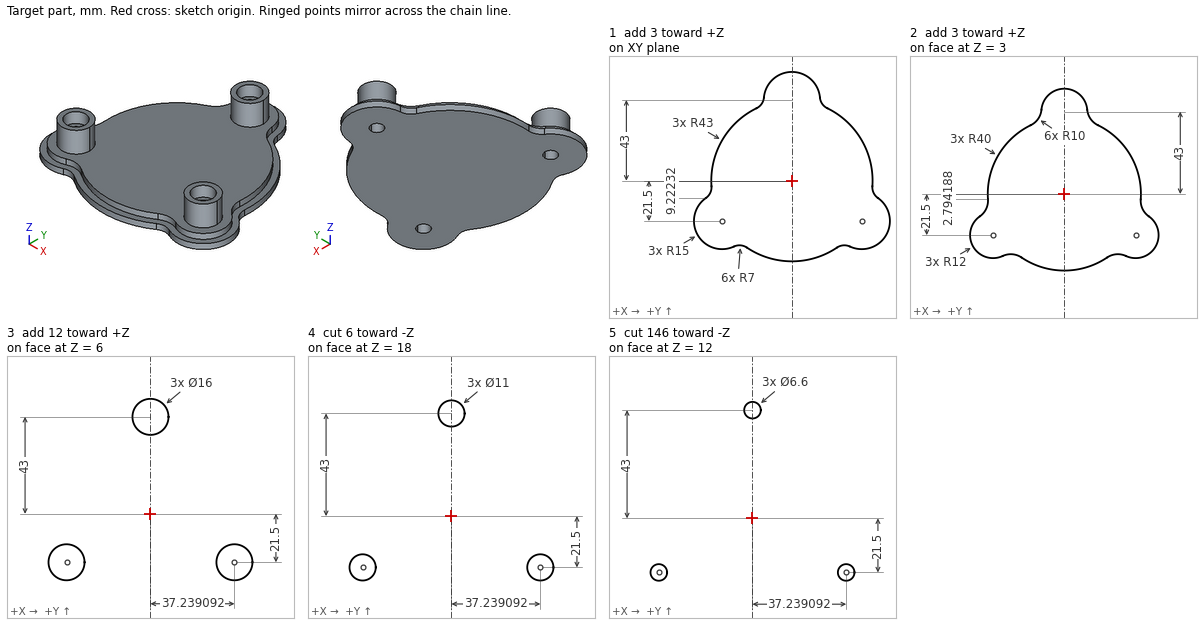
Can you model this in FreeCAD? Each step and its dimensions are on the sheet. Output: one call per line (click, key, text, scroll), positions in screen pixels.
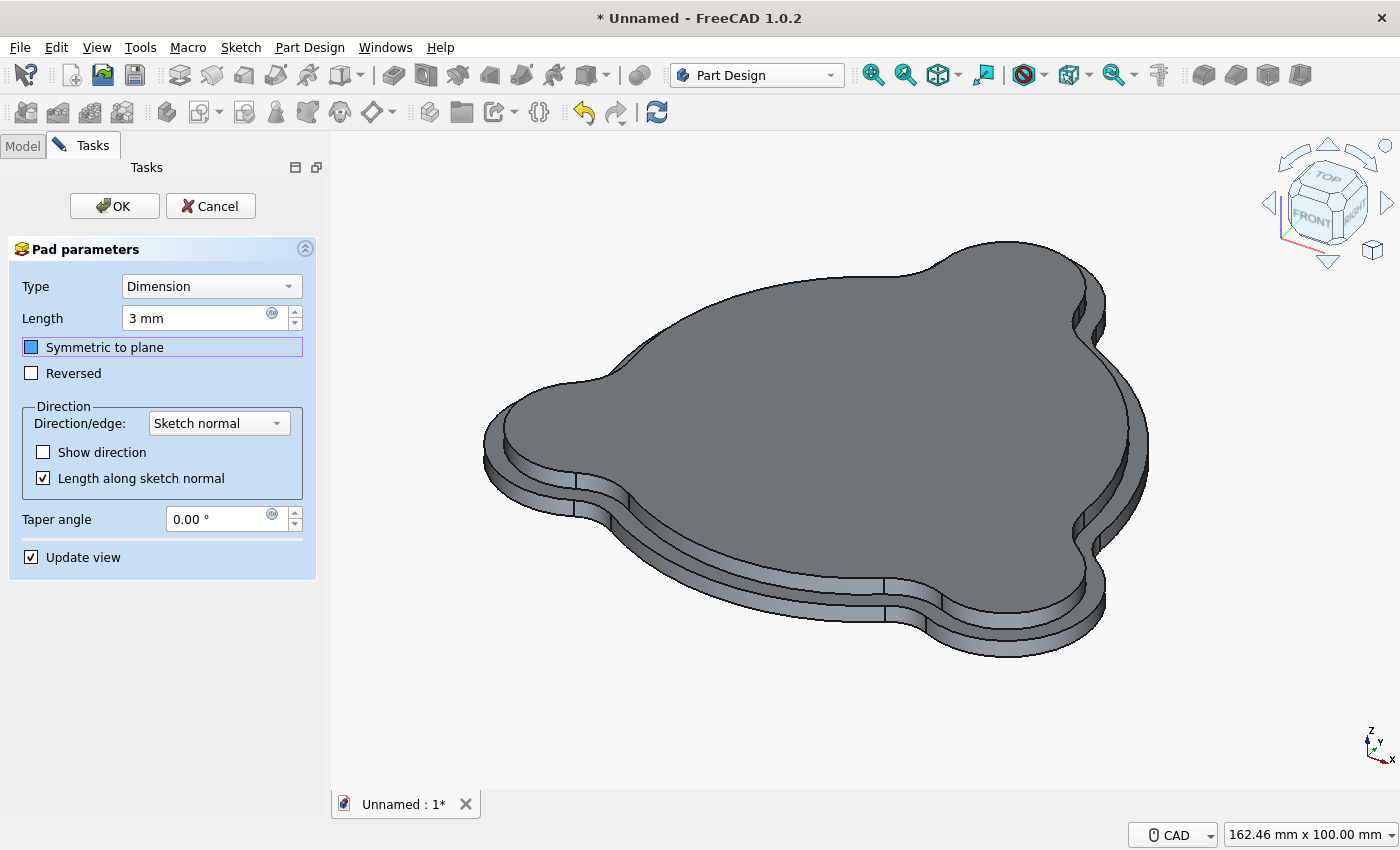
click(115, 206)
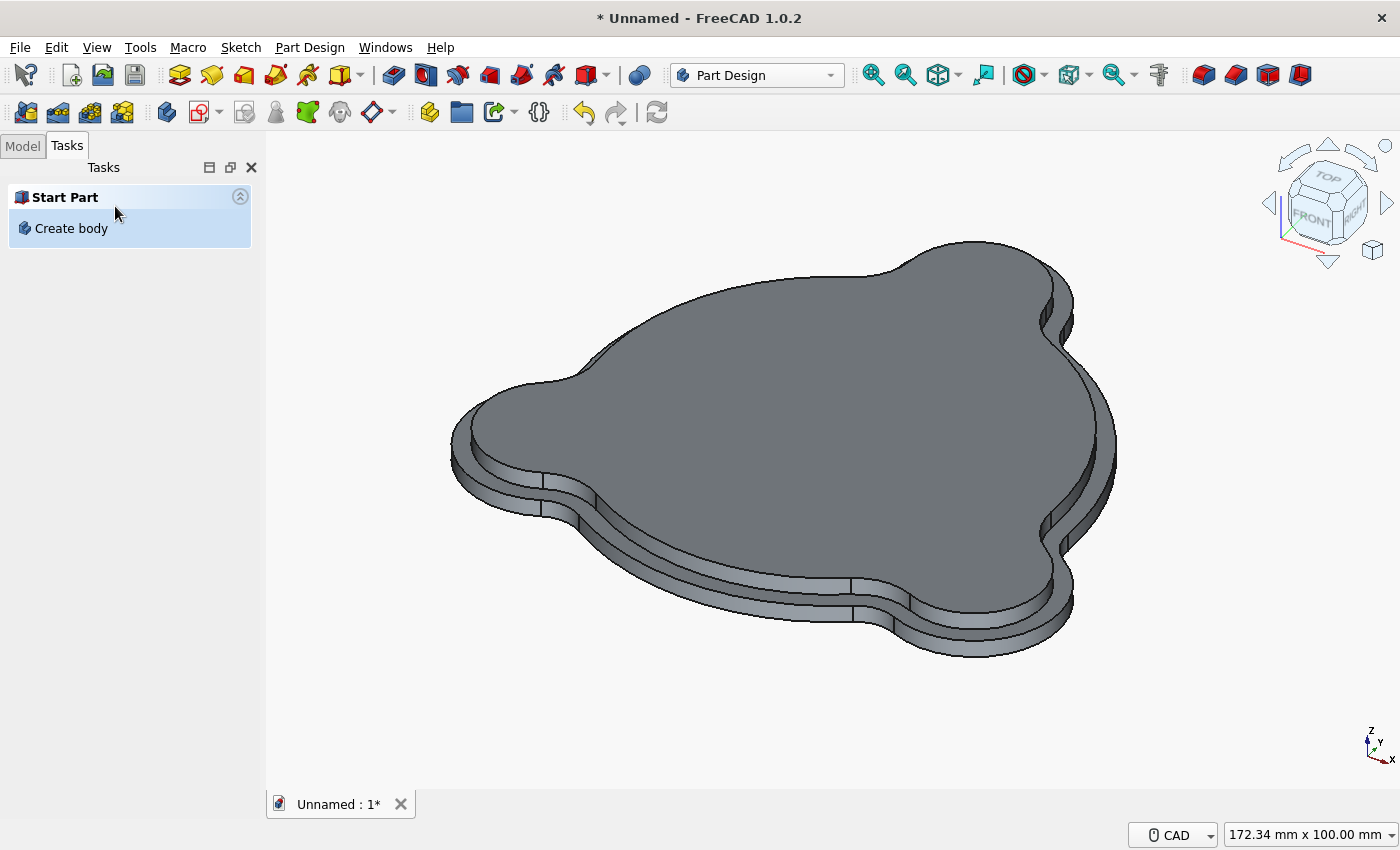
click(813, 447)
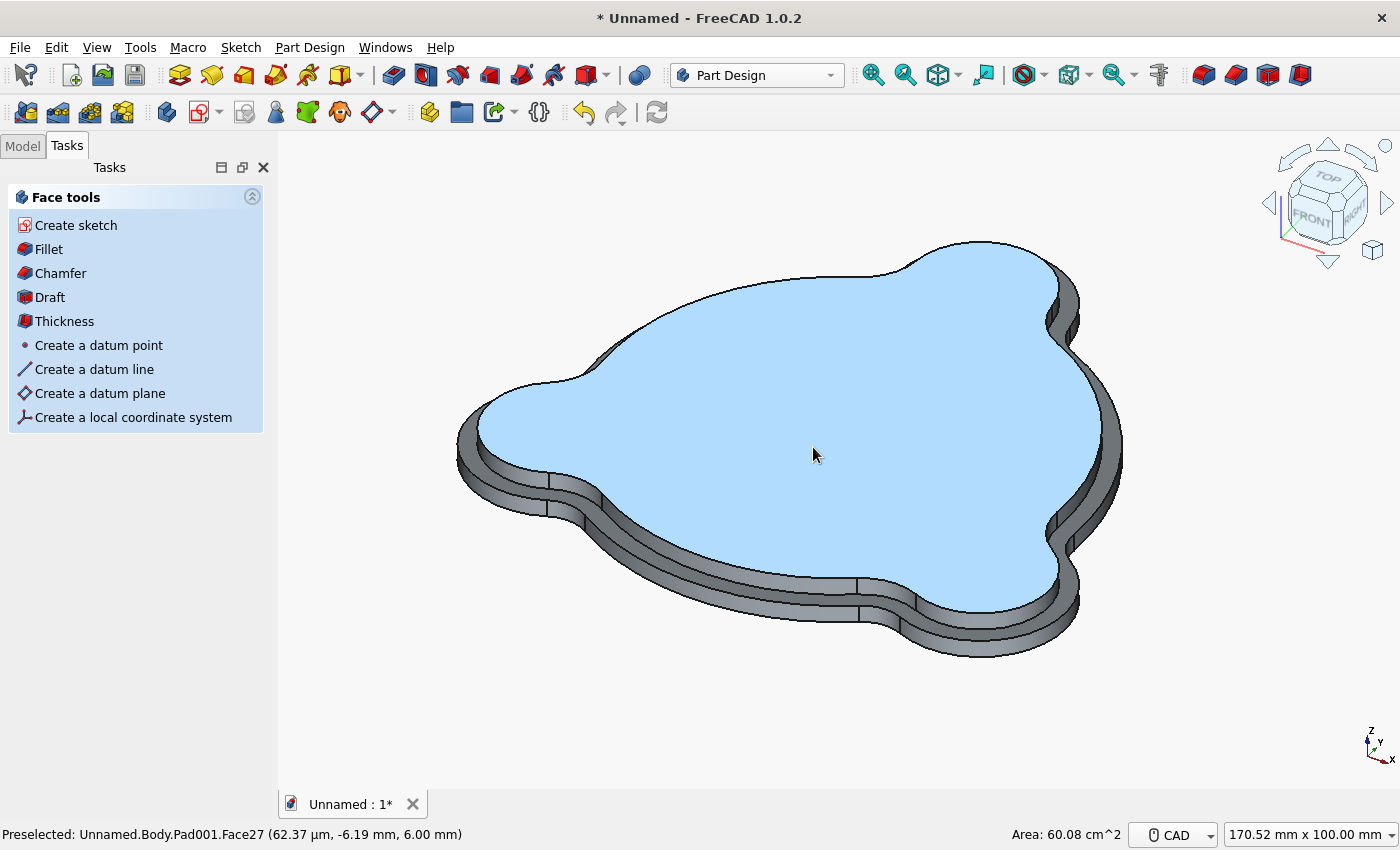
click(200, 112)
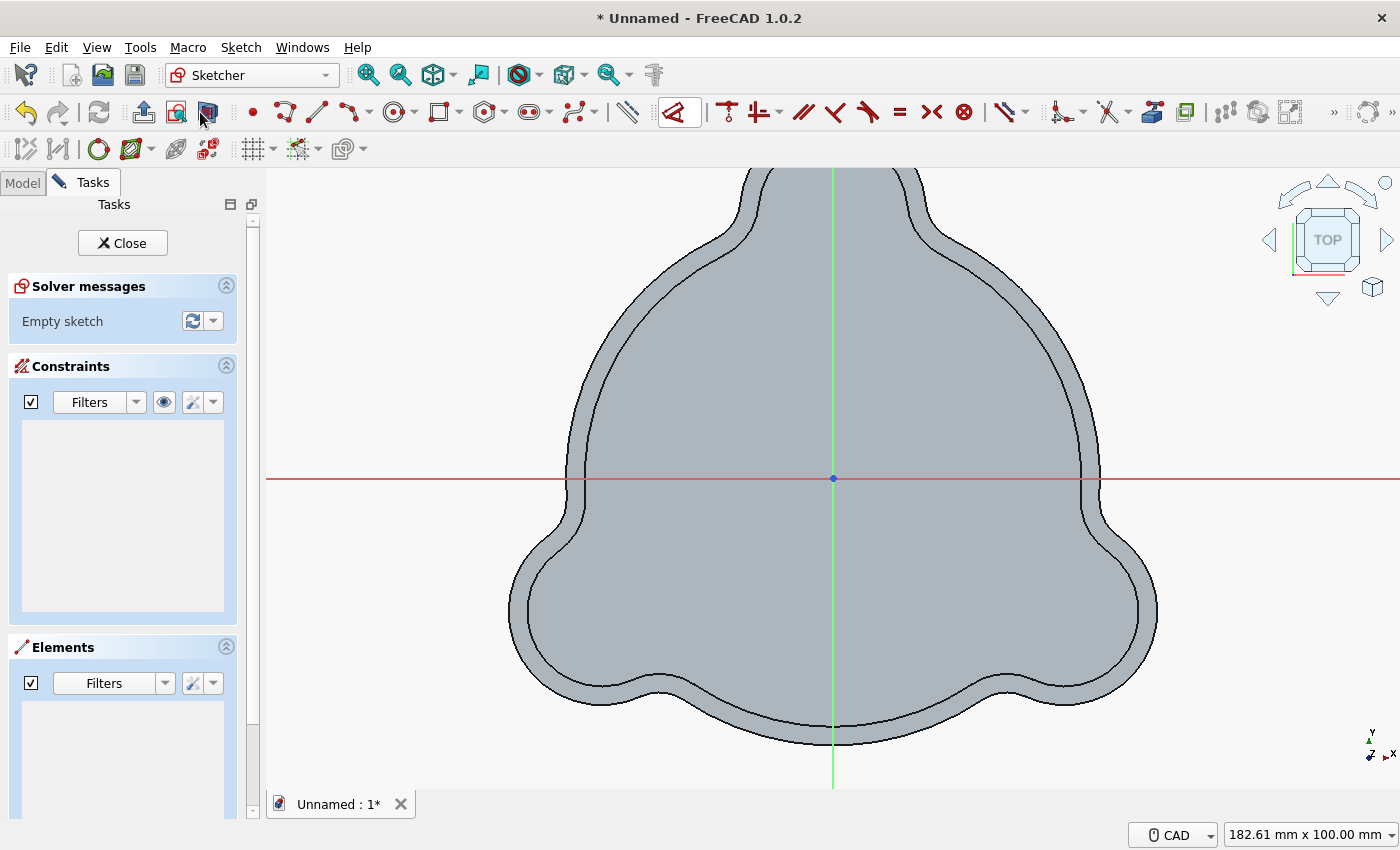
scroll(455, 761, down, 1)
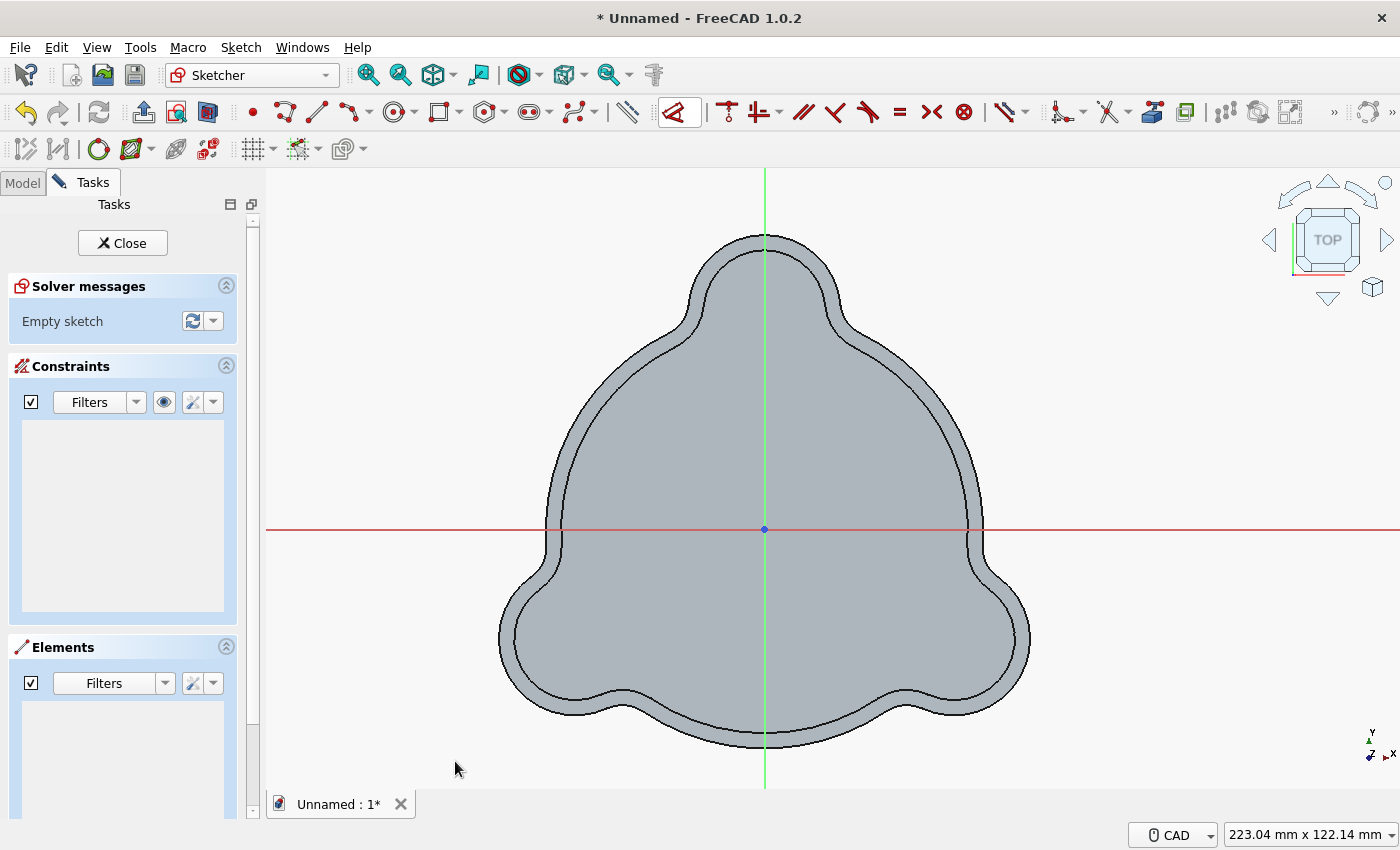
click(394, 112)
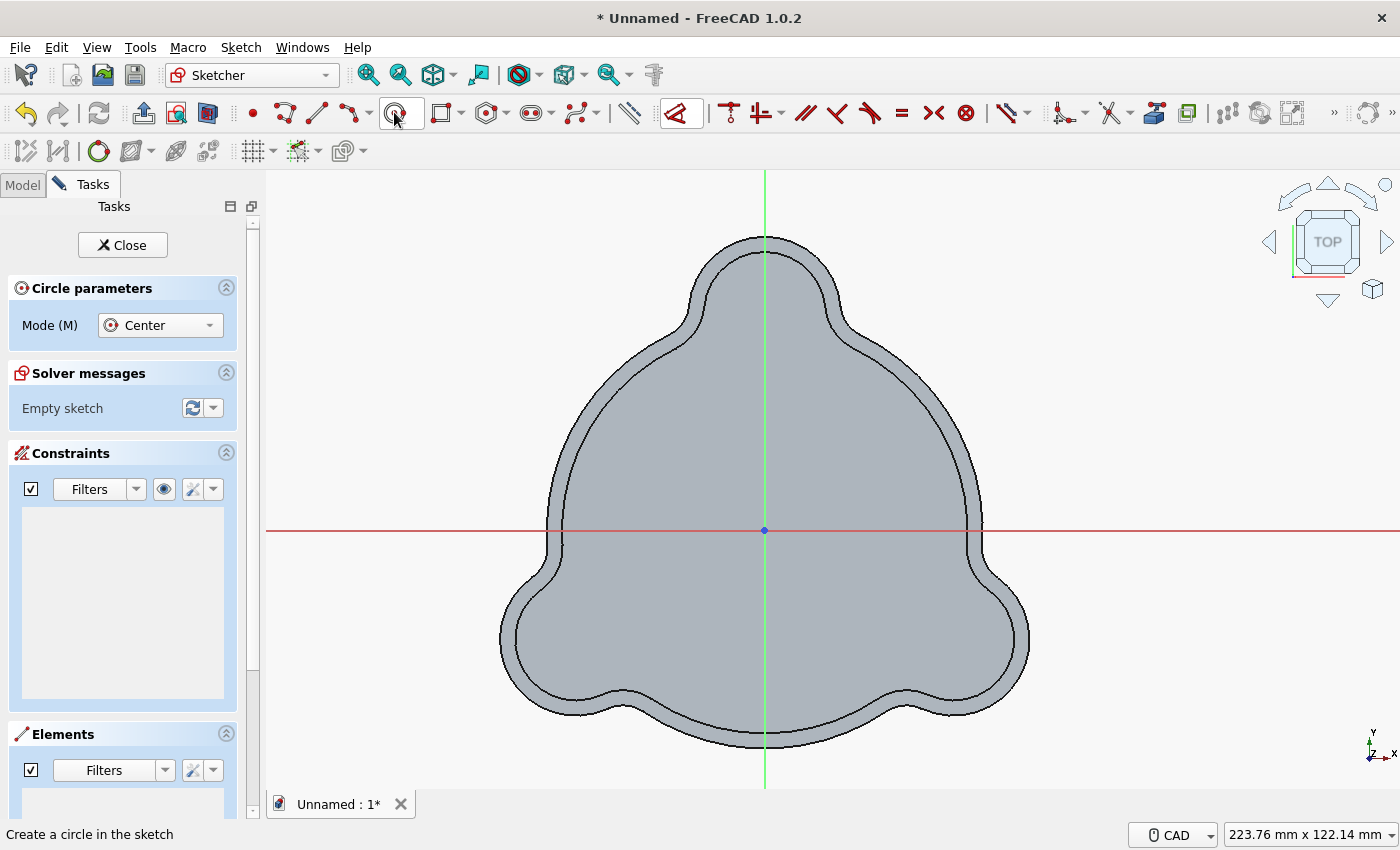
click(765, 313)
move(793, 284)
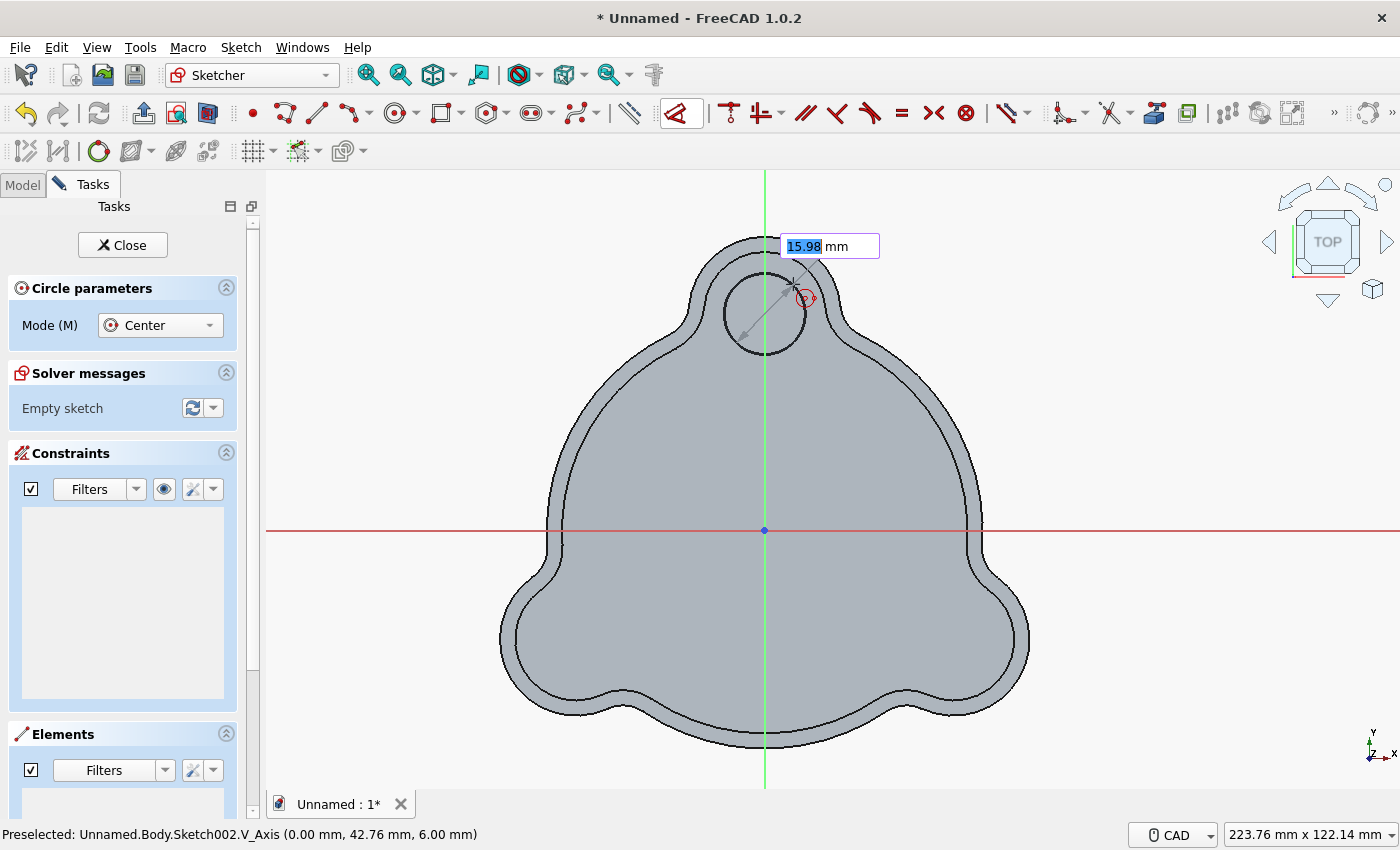
text(16)
key(Return)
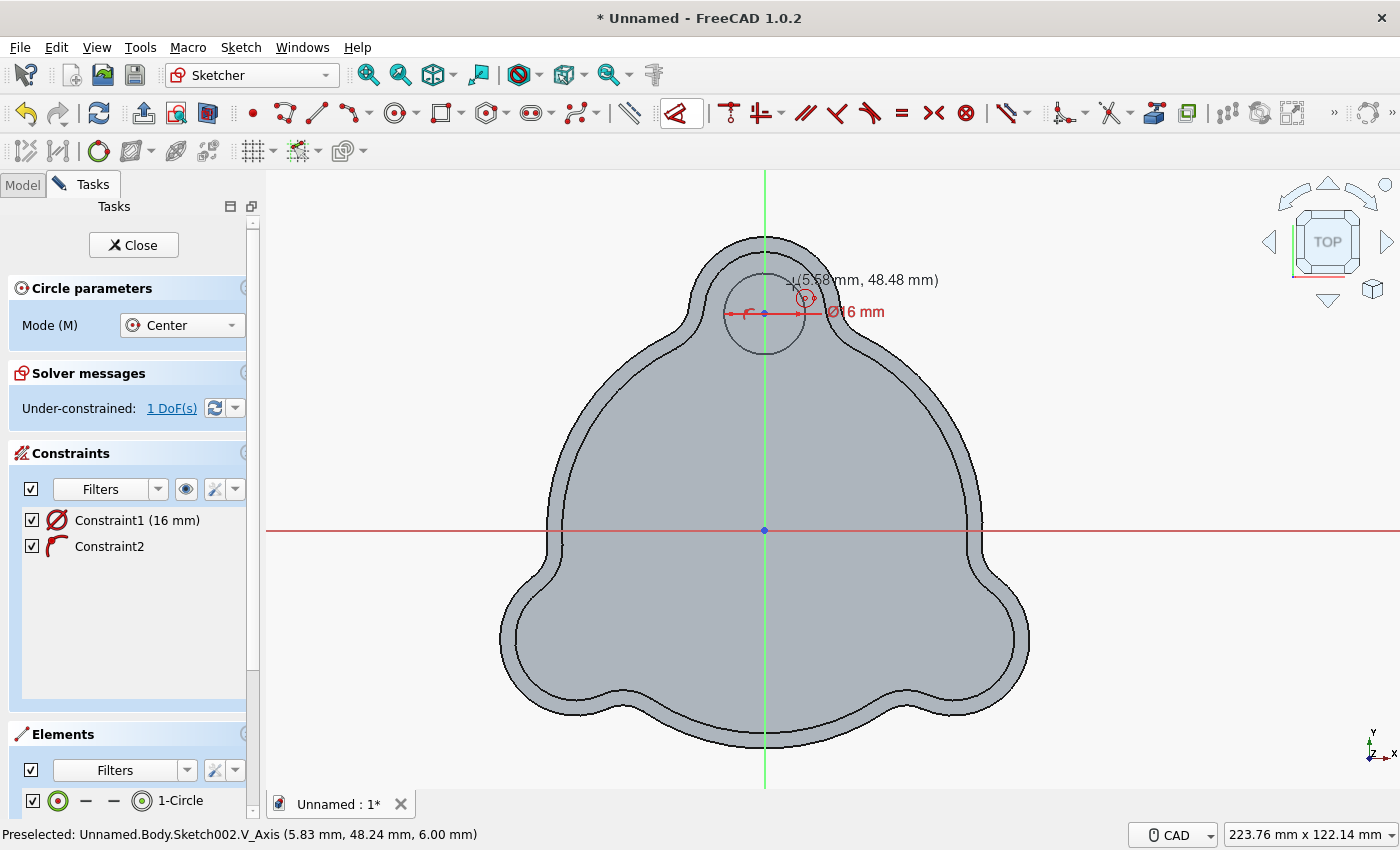
click(953, 640)
move(982, 611)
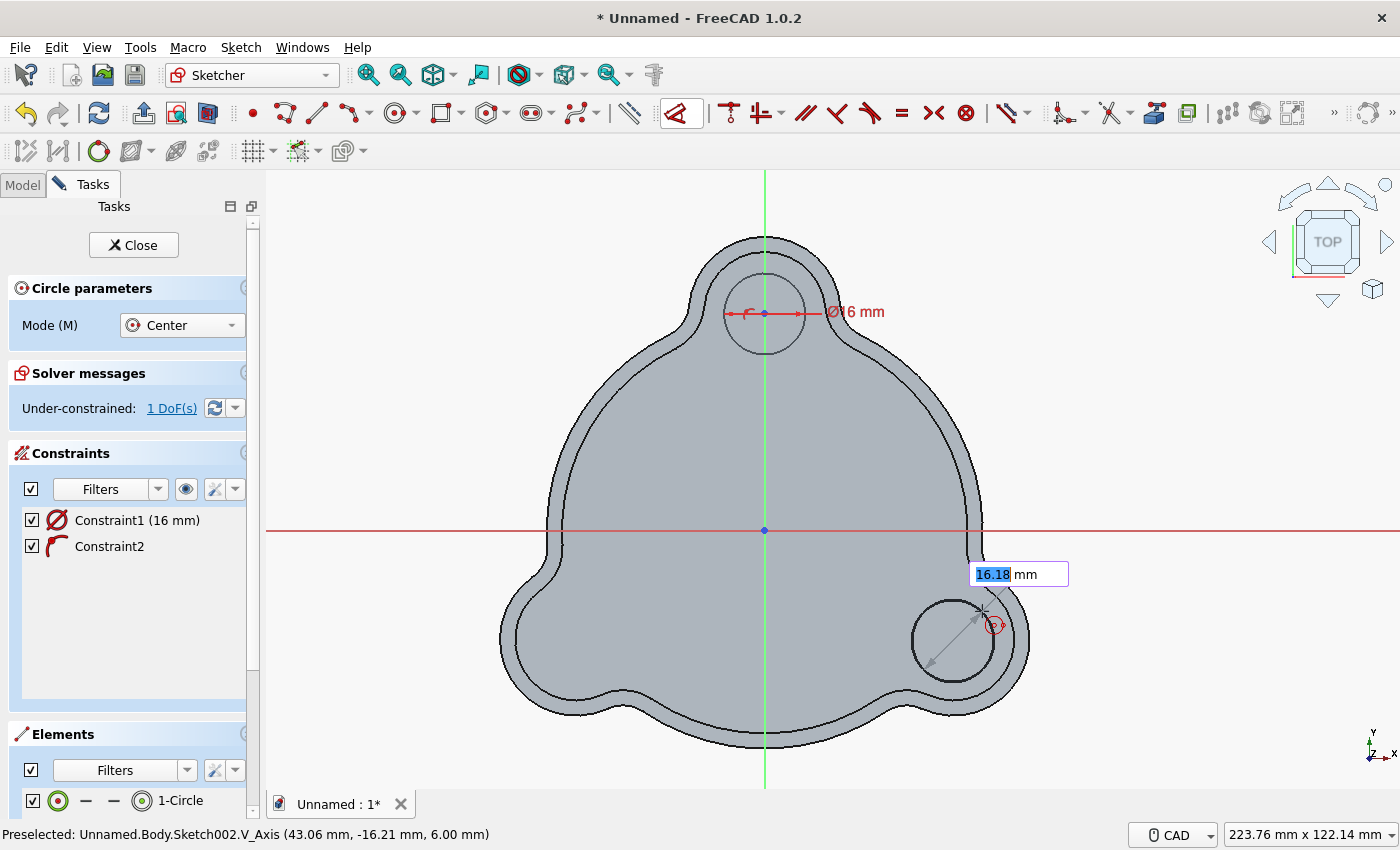
text(16)
key(Return)